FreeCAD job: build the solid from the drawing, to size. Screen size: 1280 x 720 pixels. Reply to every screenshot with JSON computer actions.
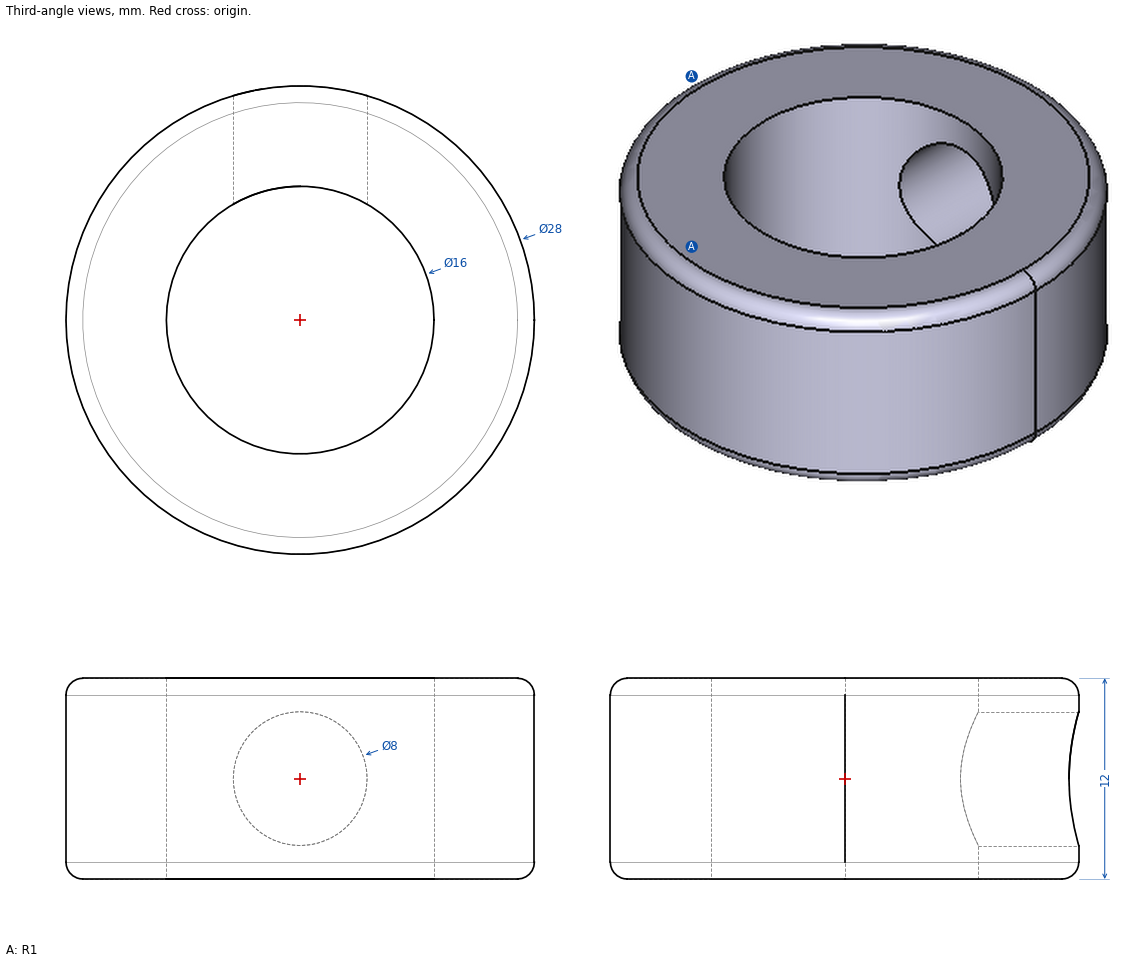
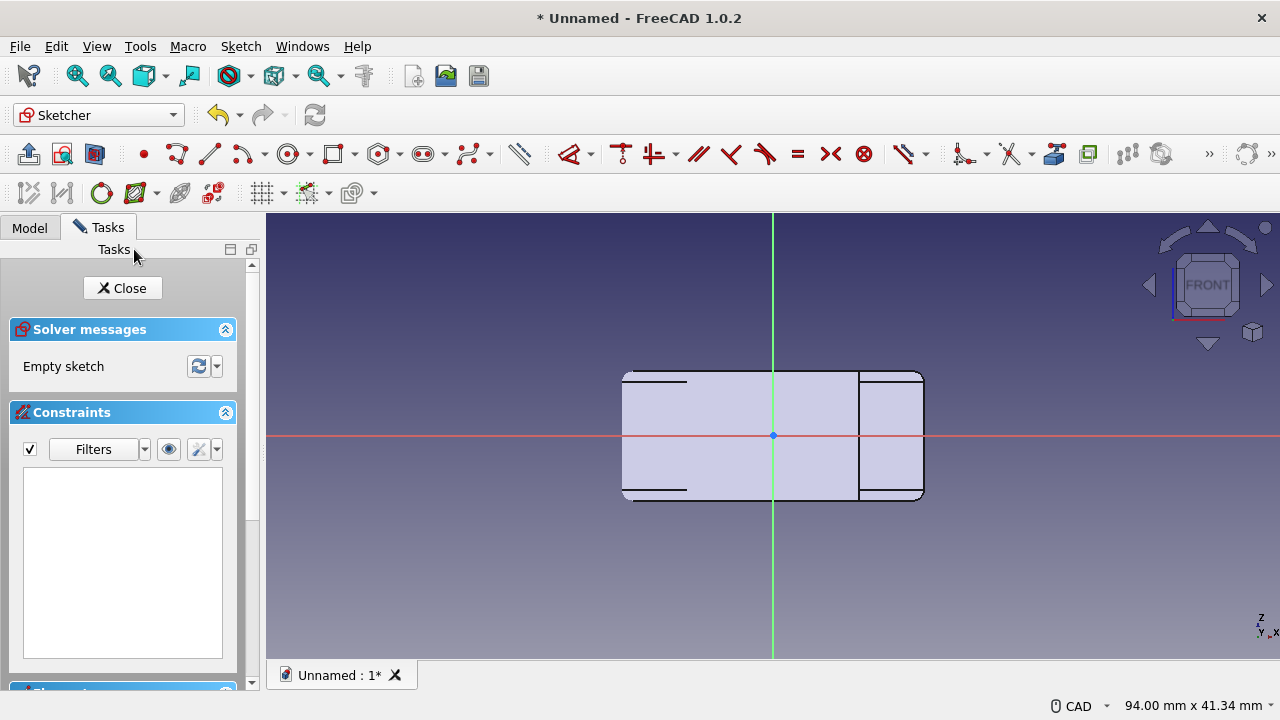
{"action": "scroll", "coordinate": [803, 436], "scroll_direction": "up", "scroll_amount": 6}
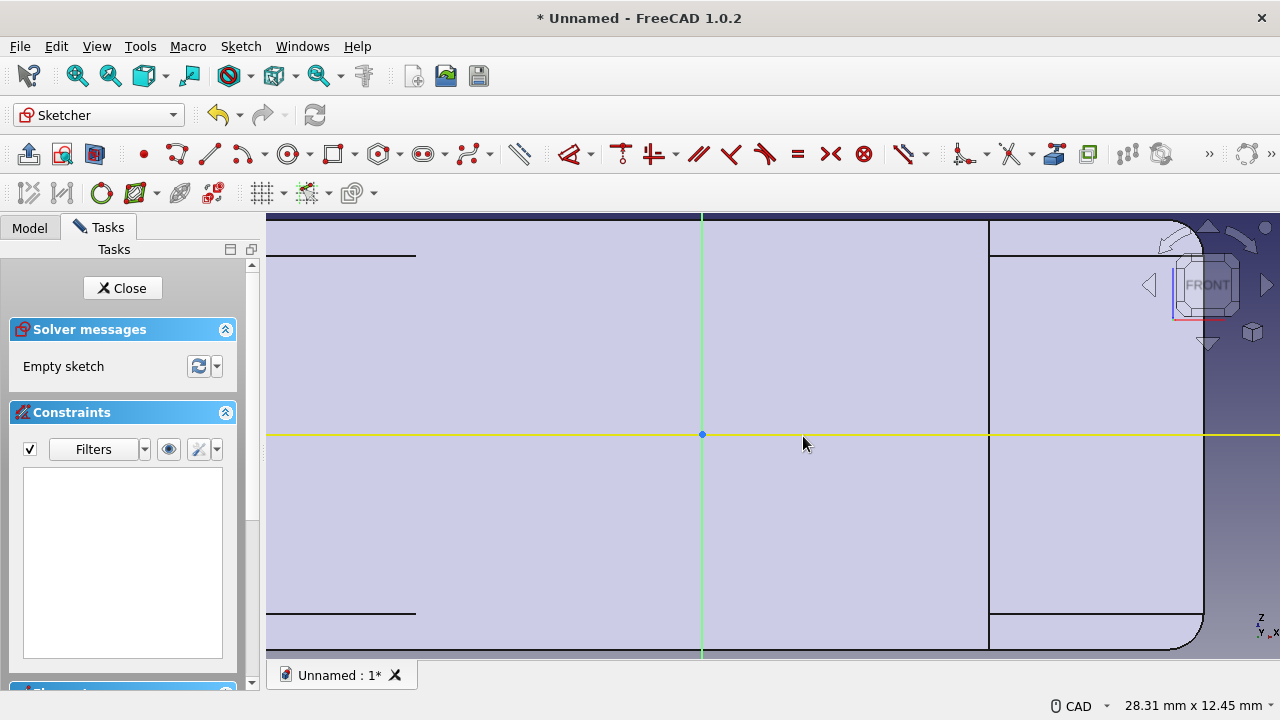
{"action": "key", "text": "g c"}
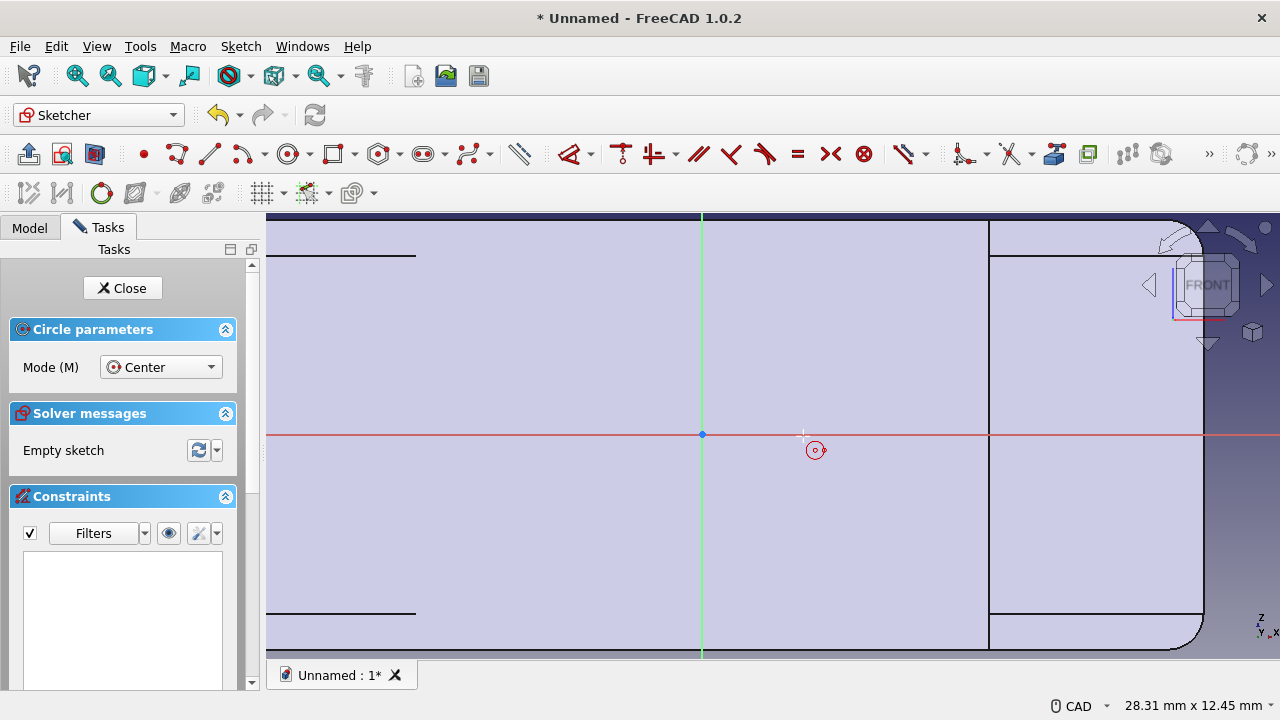
{"action": "left_click", "coordinate": [702, 435]}
{"action": "left_click", "coordinate": [803, 334]}
{"action": "key", "text": "Escape"}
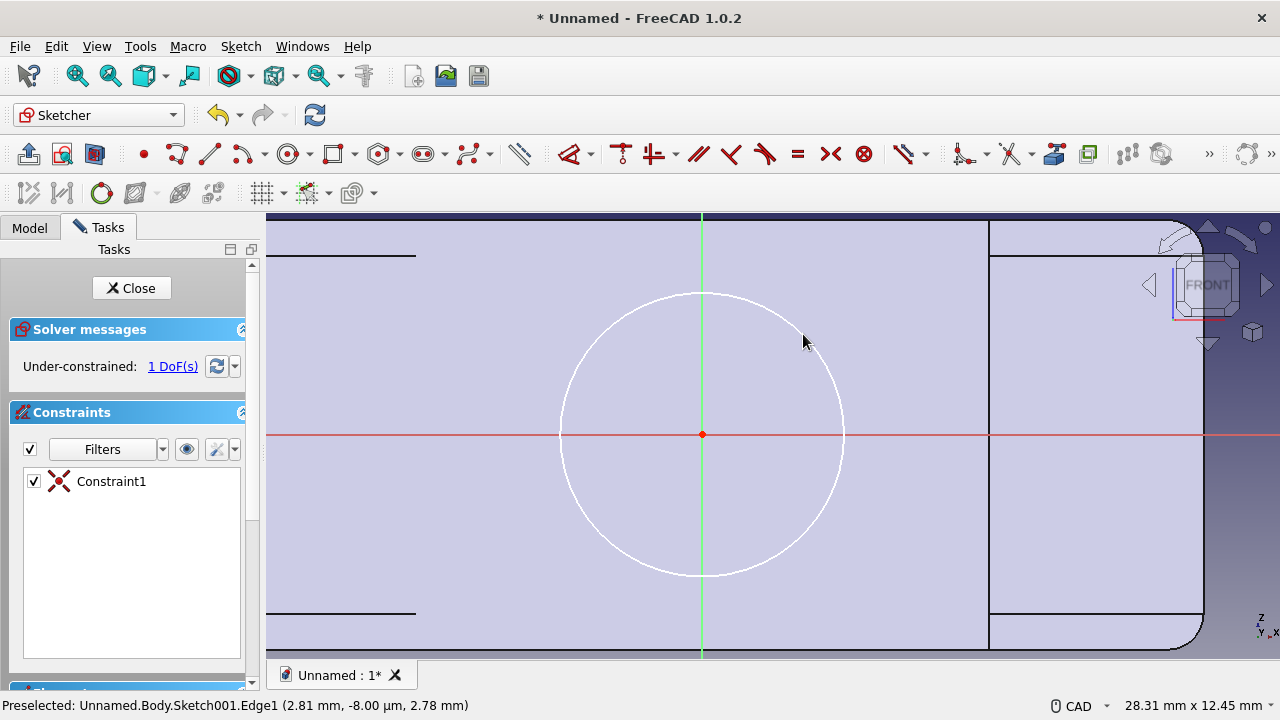
{"action": "left_click", "coordinate": [568, 154]}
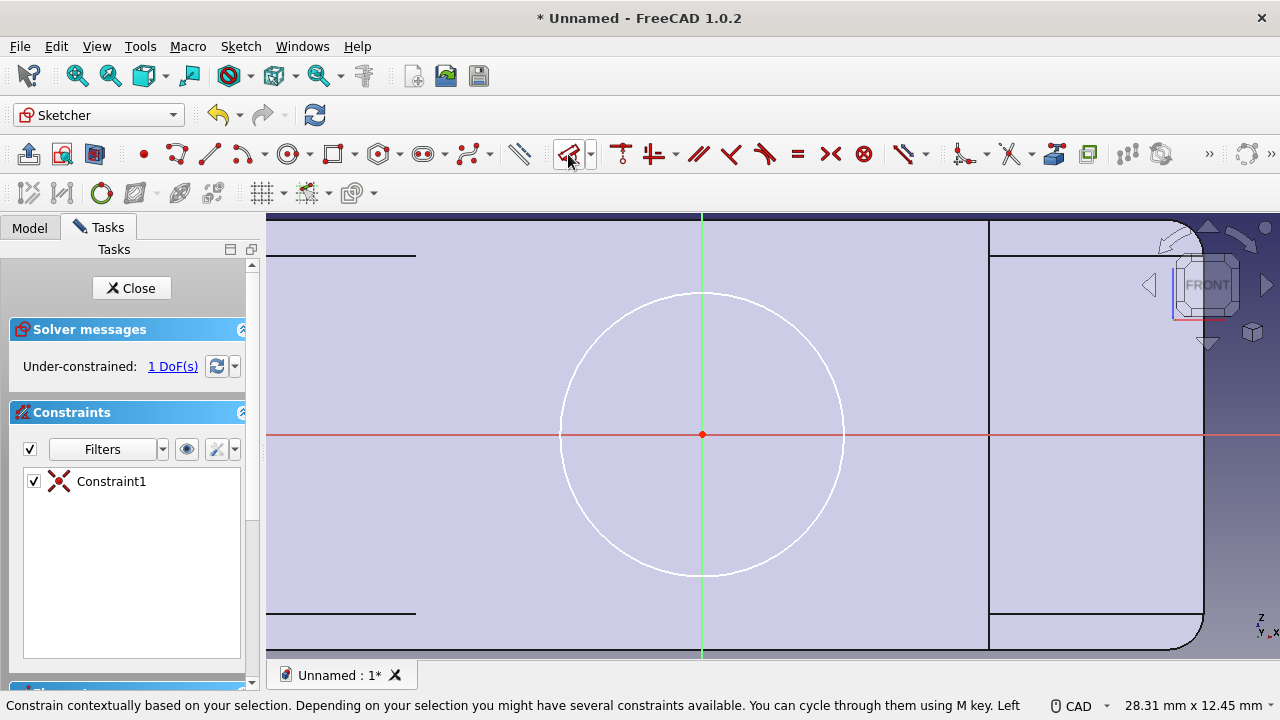
{"action": "left_click", "coordinate": [802, 334]}
{"action": "left_click", "coordinate": [825, 311]}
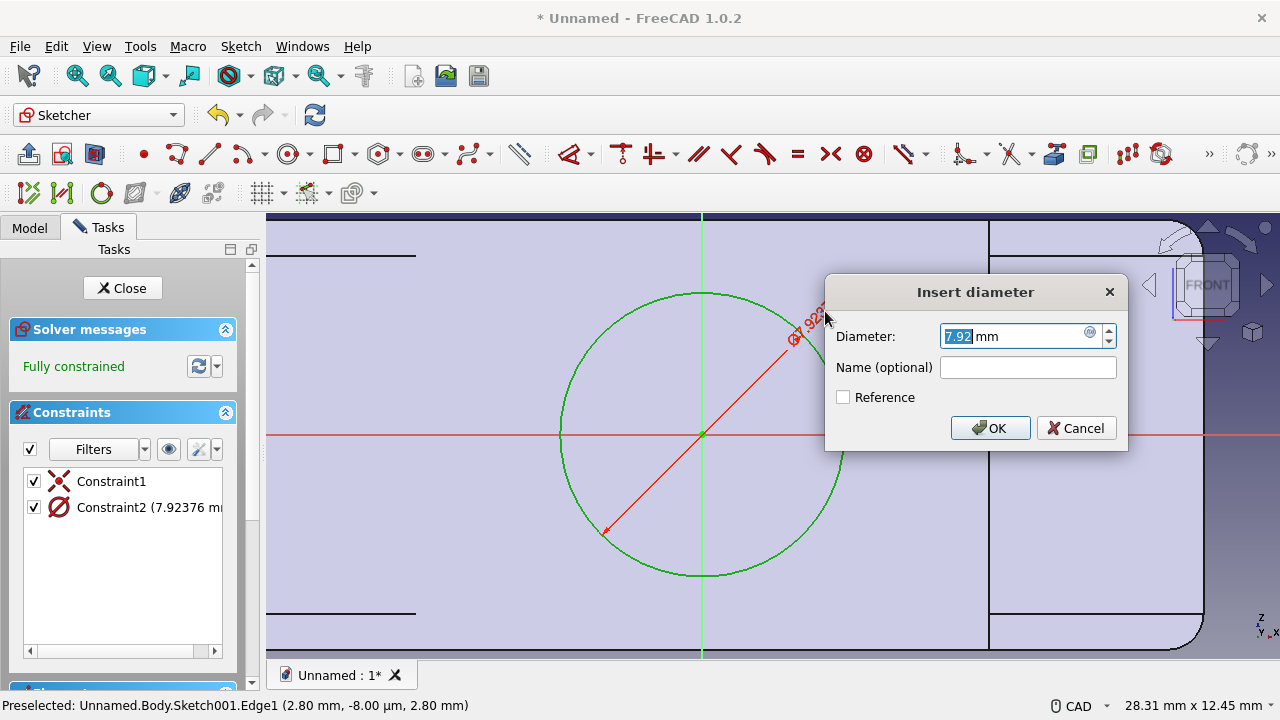
{"action": "type", "text": "8"}
{"action": "key", "text": "Return"}
{"action": "key", "text": "Escape"}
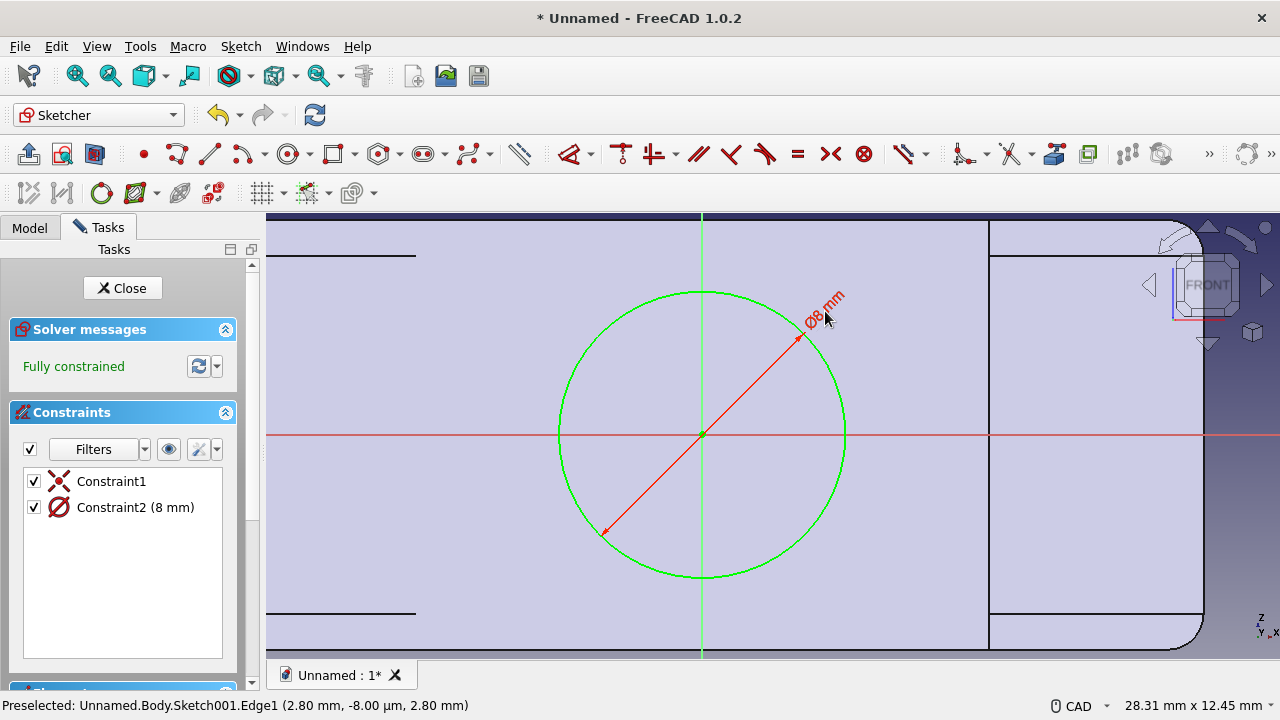
{"action": "left_click", "coordinate": [123, 288]}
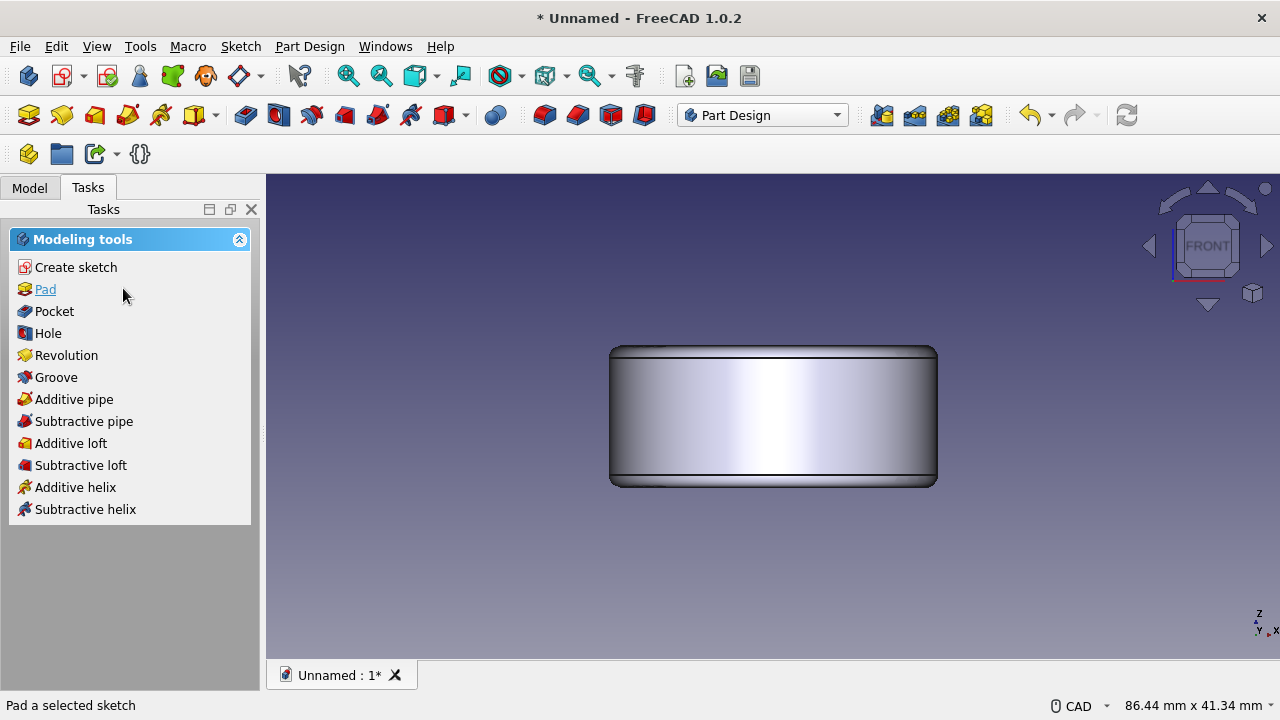
{"action": "left_click", "coordinate": [246, 116]}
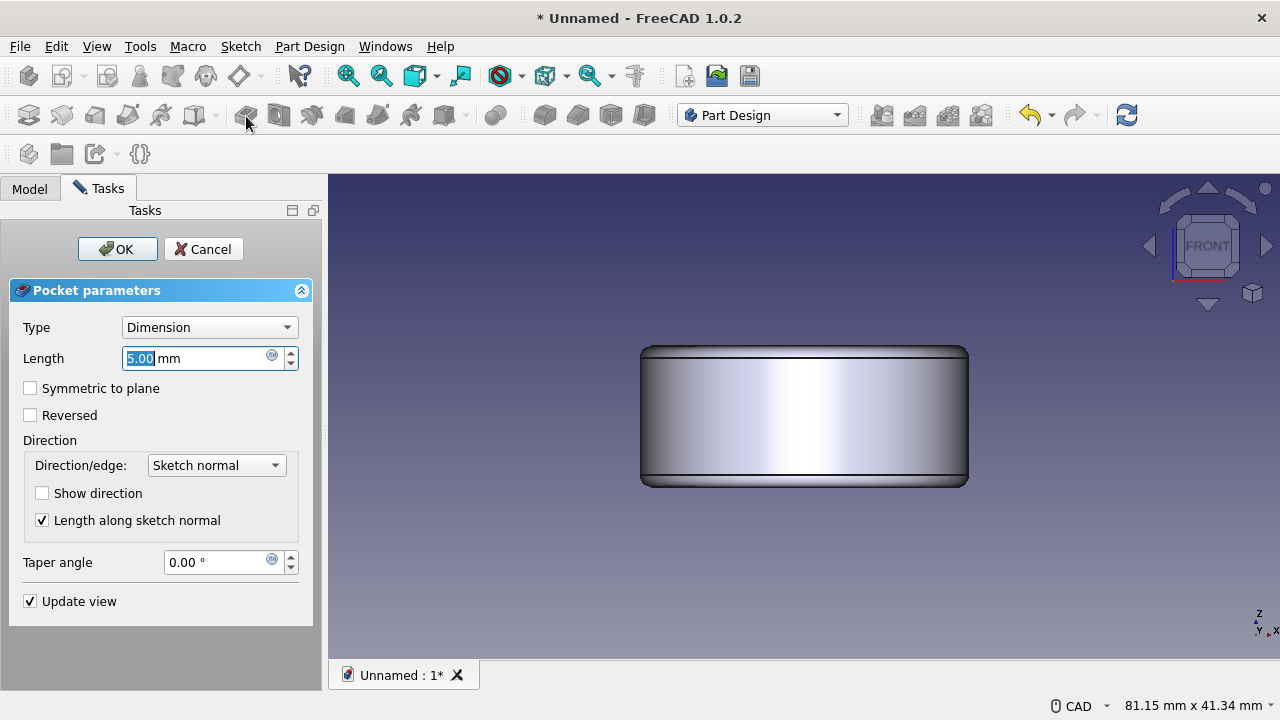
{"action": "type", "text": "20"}
{"action": "key", "text": "Tab"}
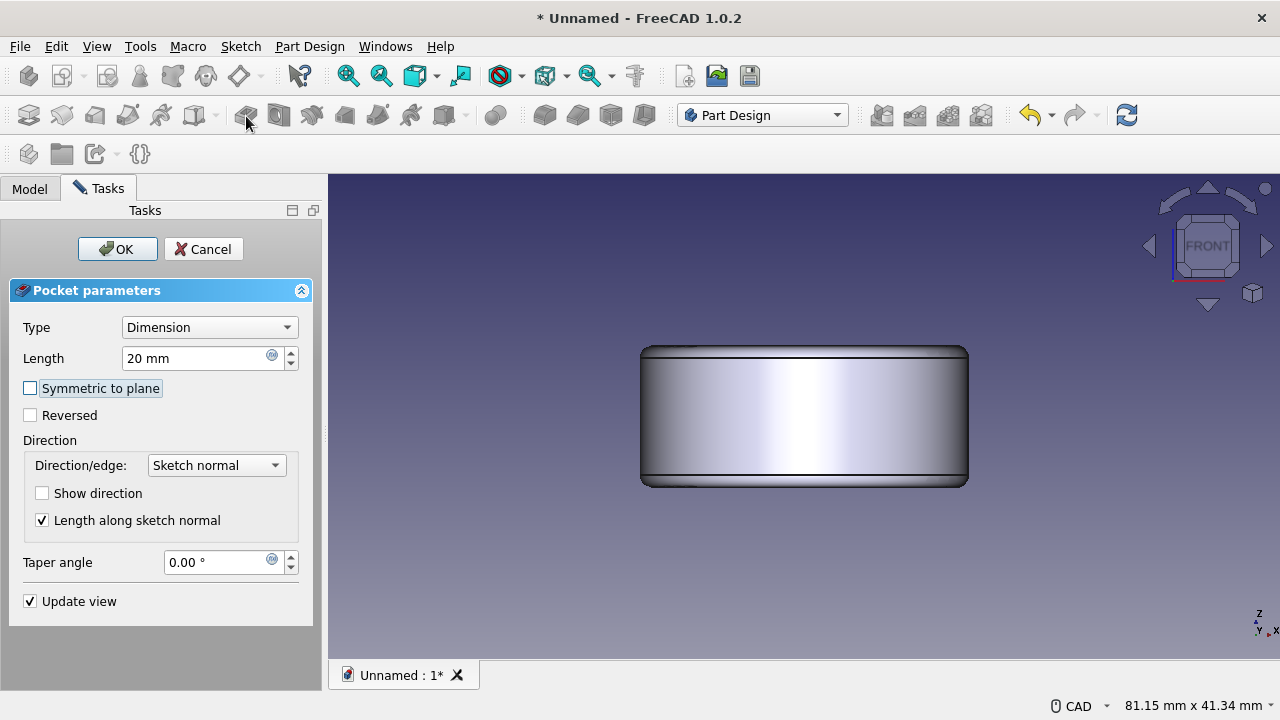
{"action": "left_click", "coordinate": [118, 249]}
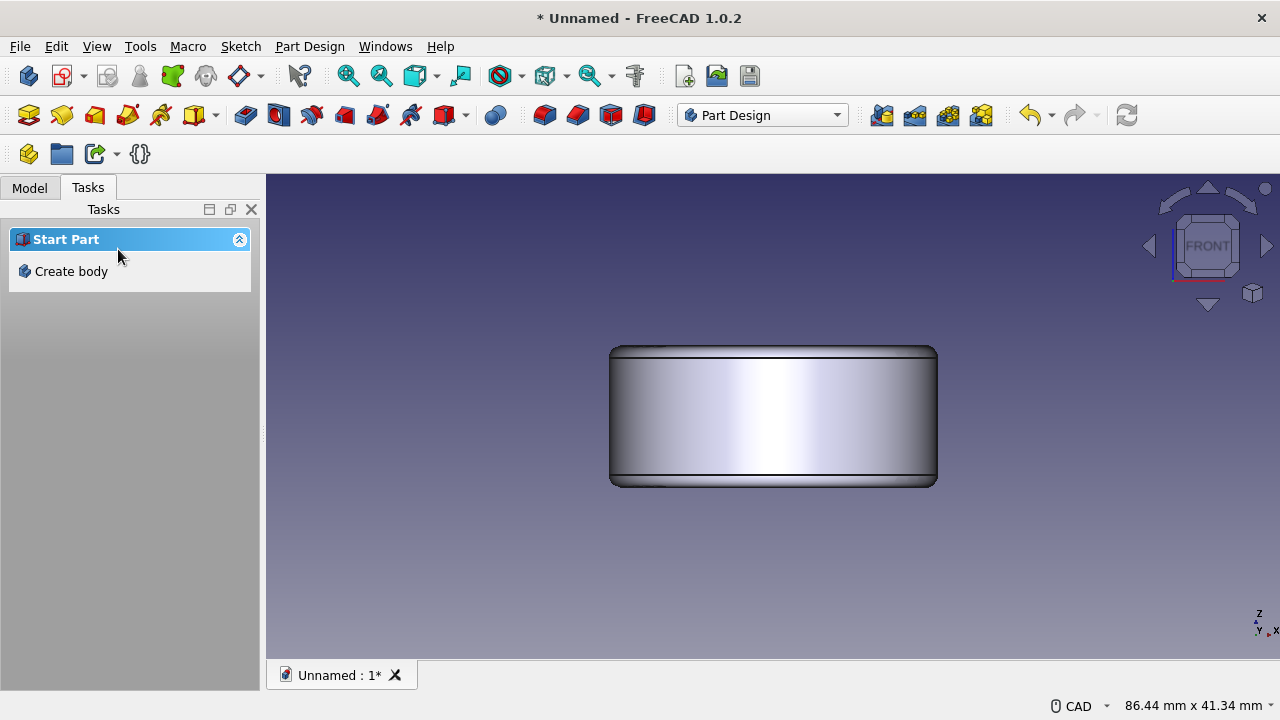
{"action": "key", "text": "0"}